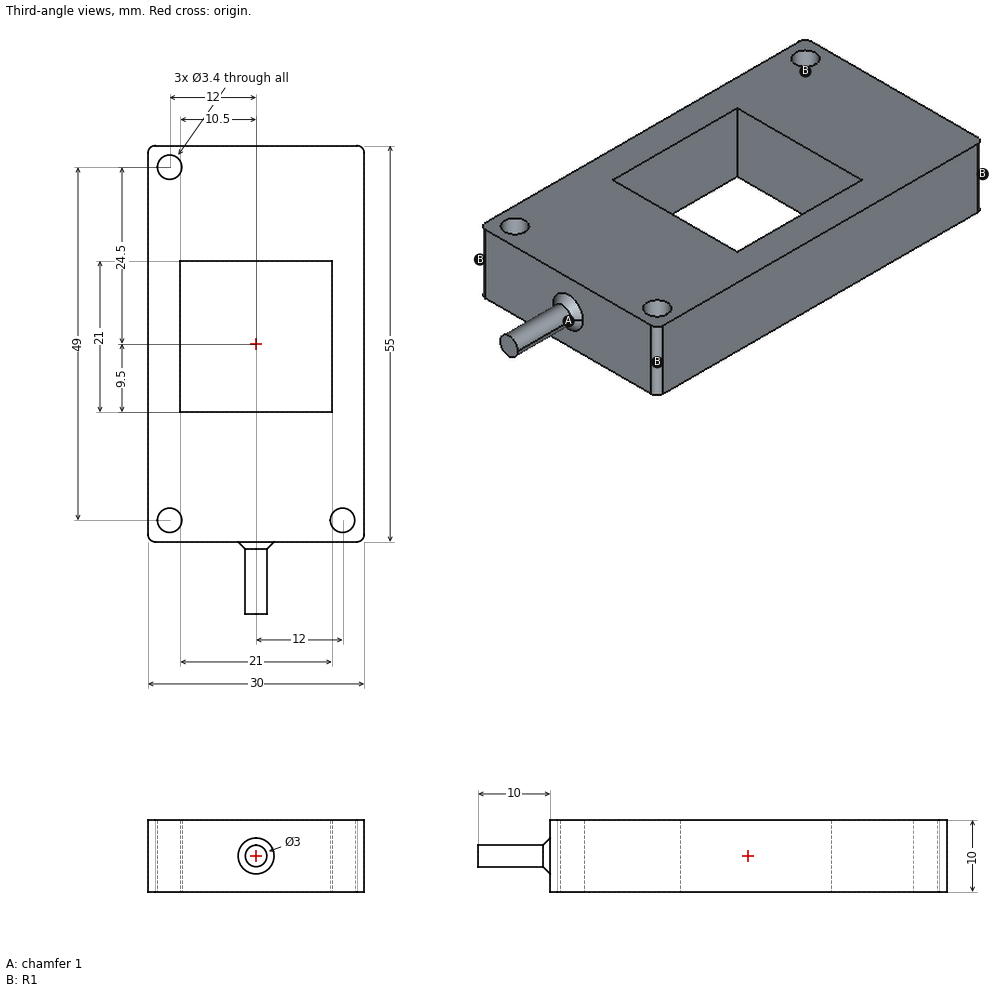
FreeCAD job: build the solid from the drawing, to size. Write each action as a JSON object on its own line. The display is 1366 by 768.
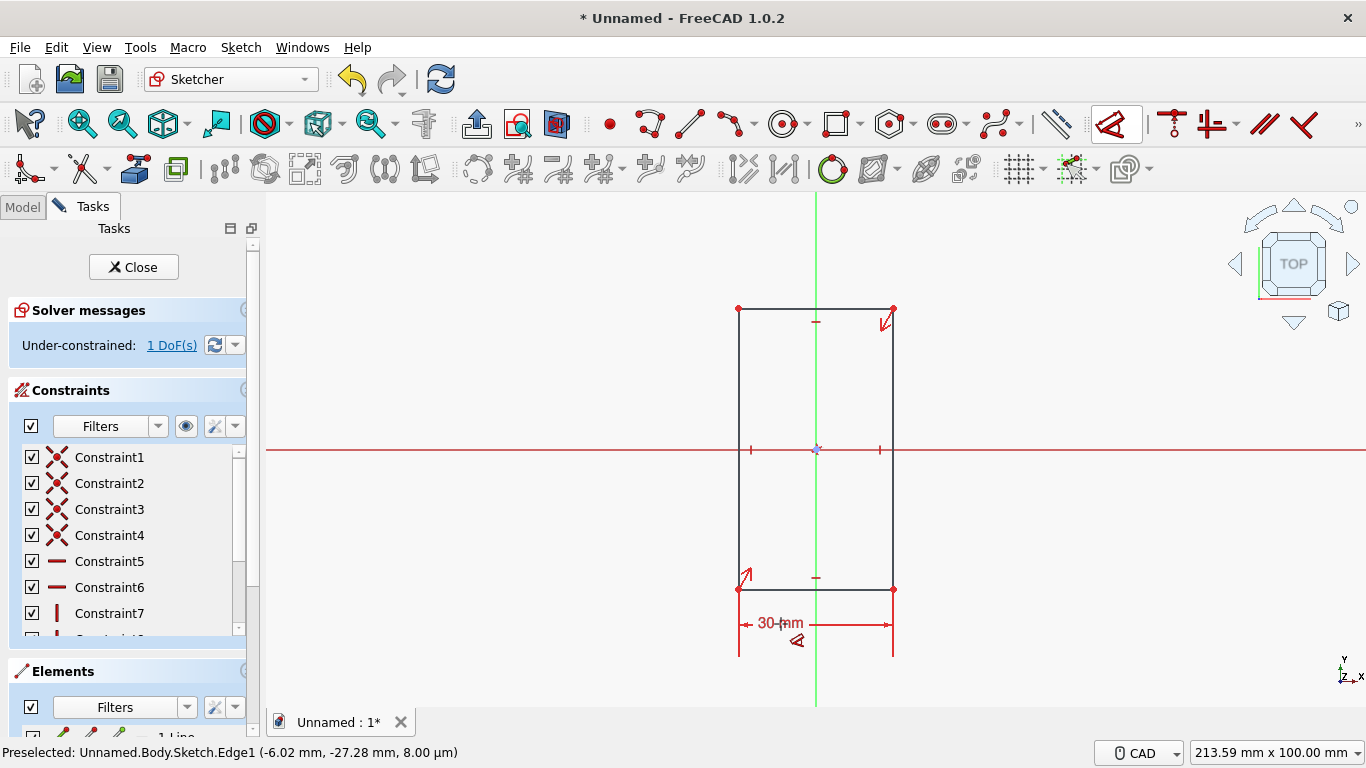
{"action": "left_click", "coordinate": [893, 506]}
{"action": "left_click", "coordinate": [927, 385]}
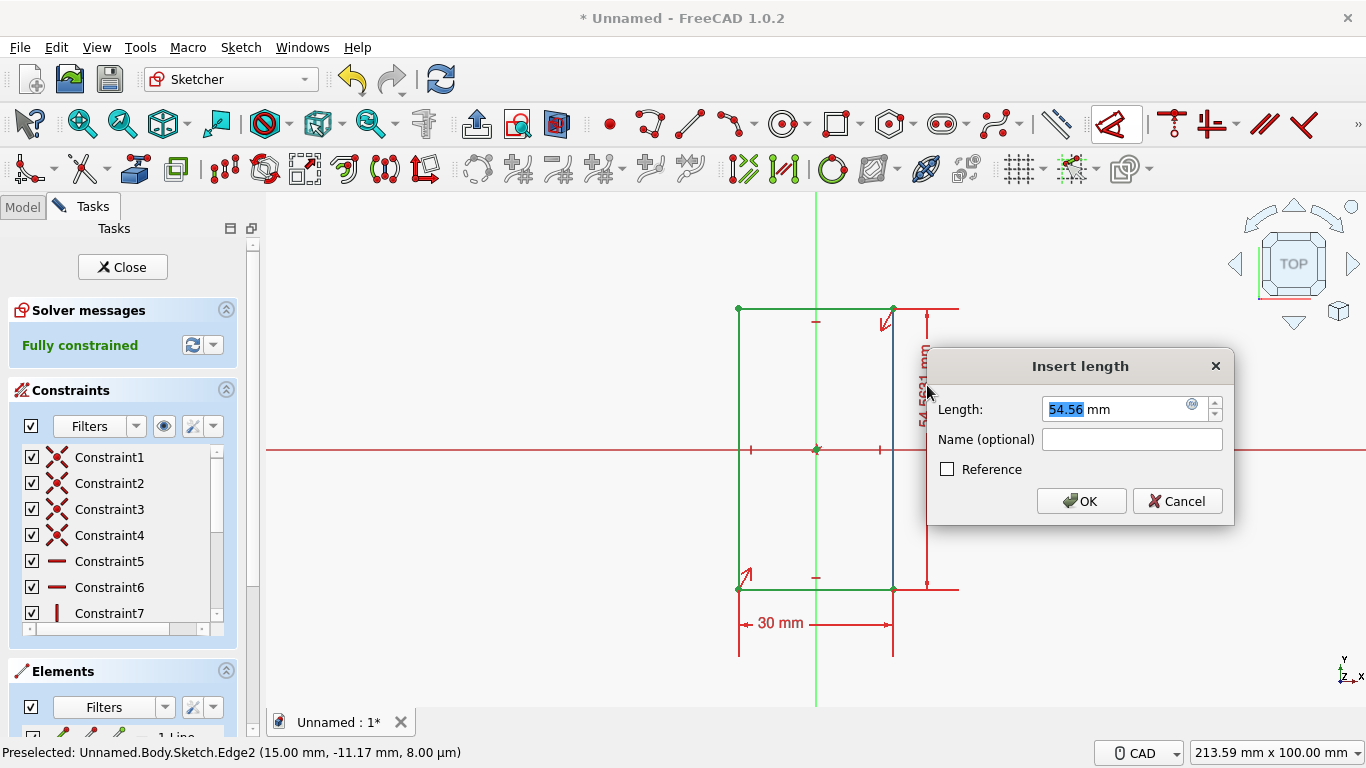
{"action": "type", "text": "55"}
{"action": "key", "text": "Return"}
{"action": "key", "text": "Escape"}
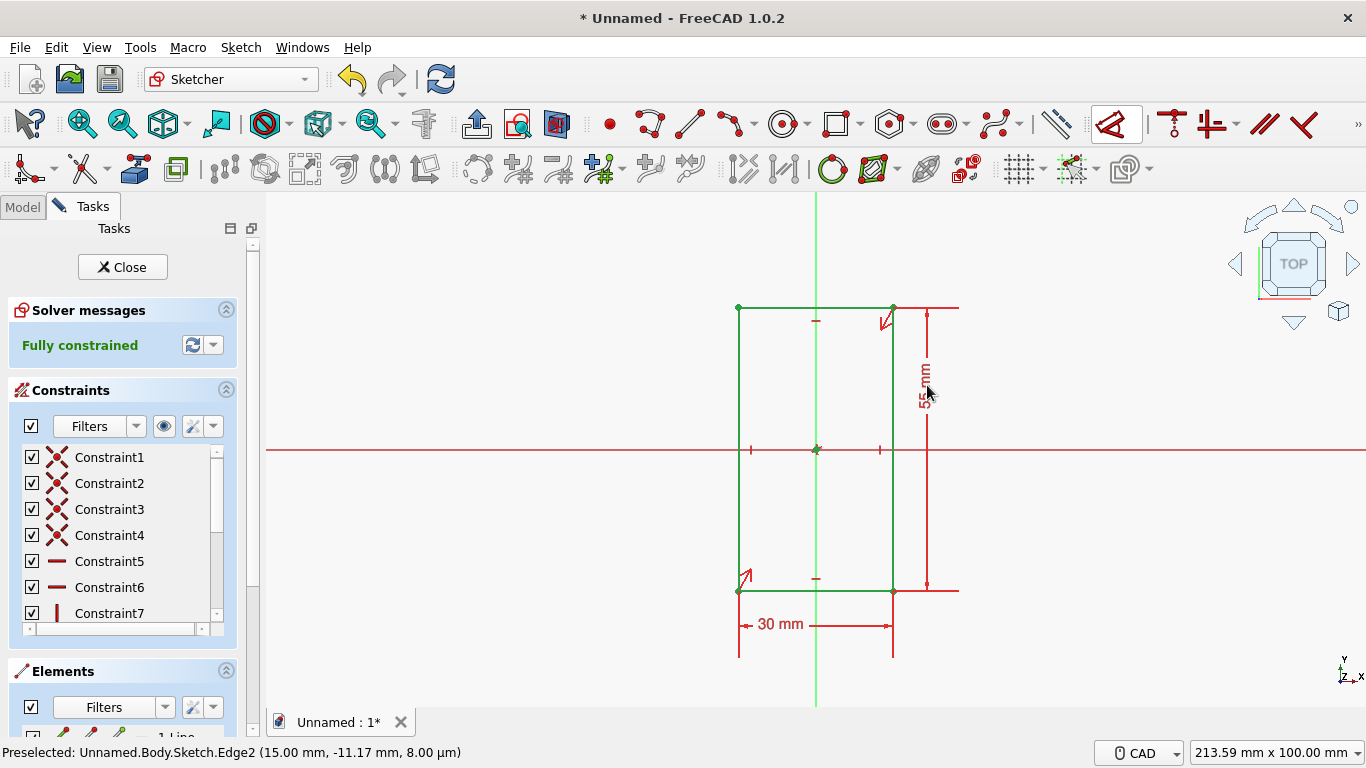
{"action": "left_click", "coordinate": [123, 267]}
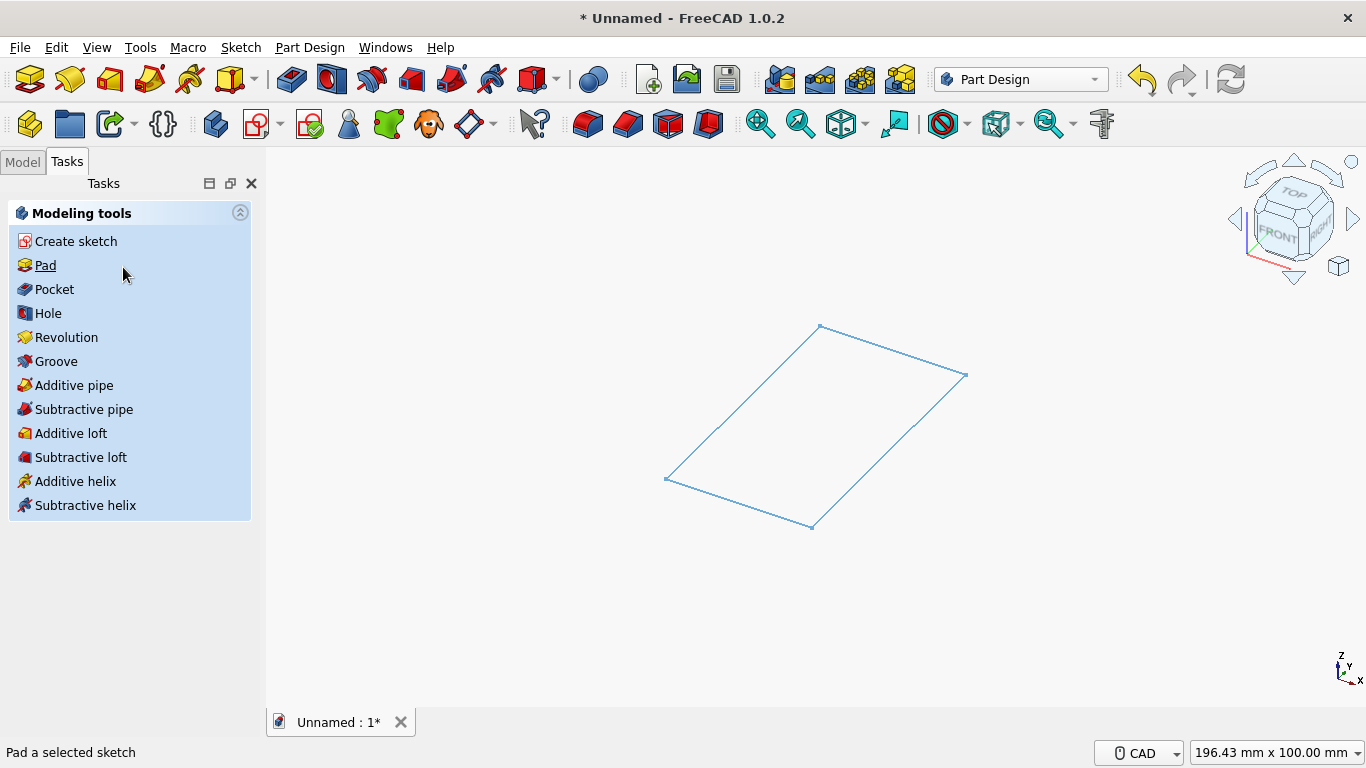
{"action": "left_click", "coordinate": [30, 80]}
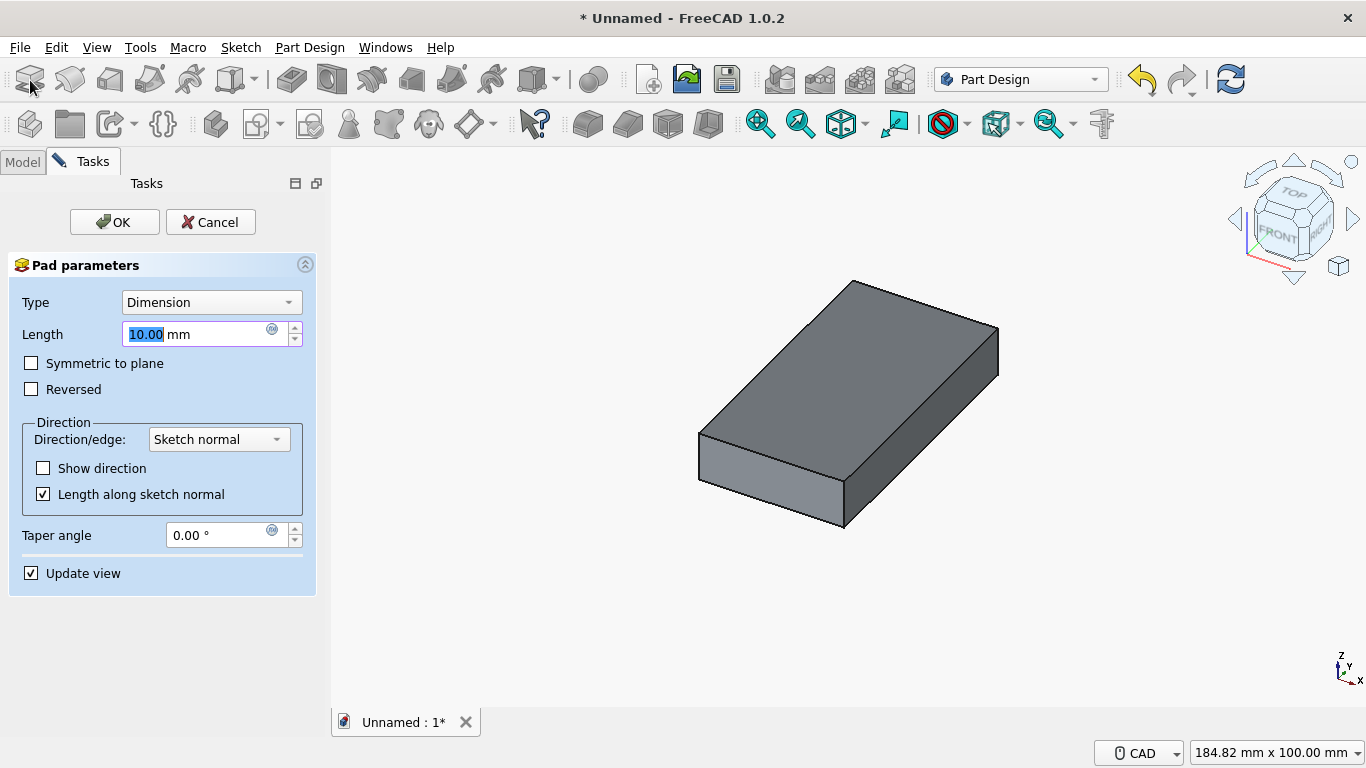
{"action": "type", "text": "10"}
{"action": "key", "text": "Tab"}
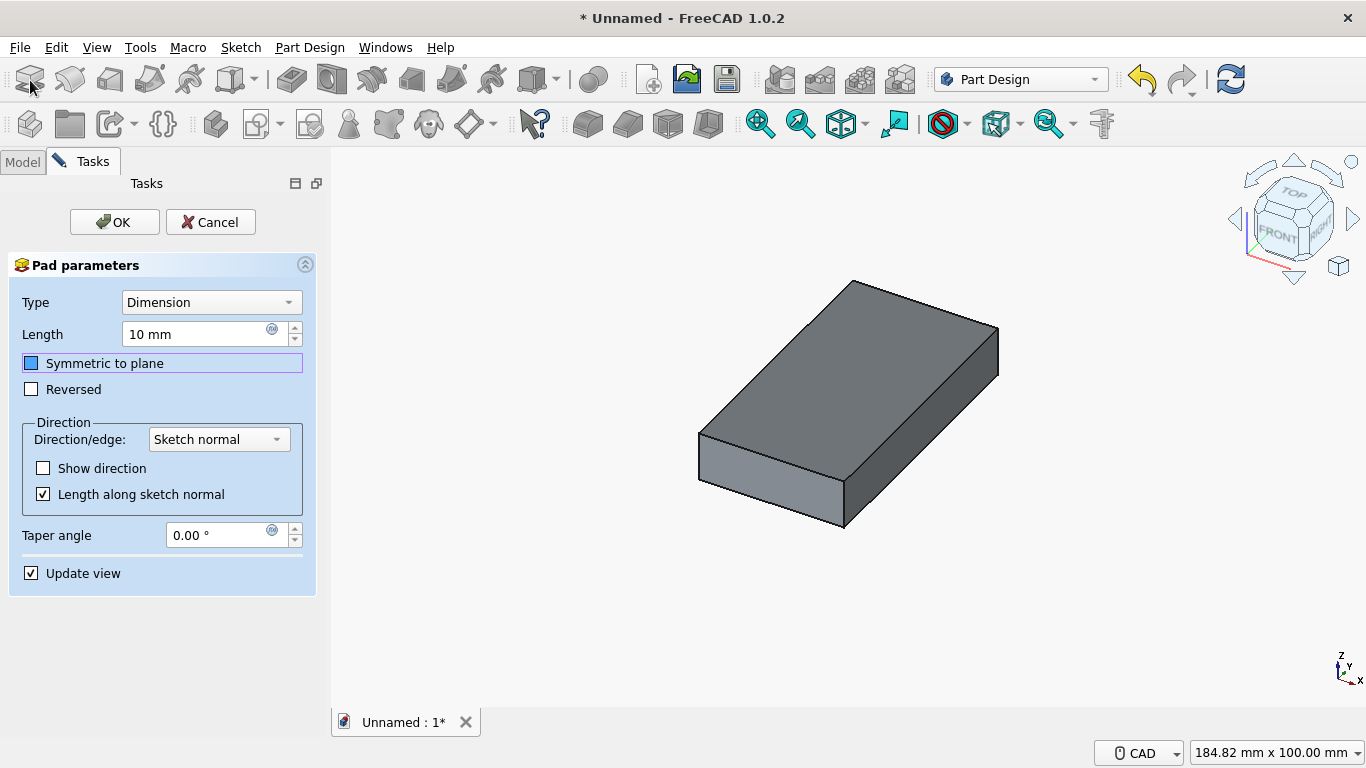
{"action": "left_click", "coordinate": [30, 363]}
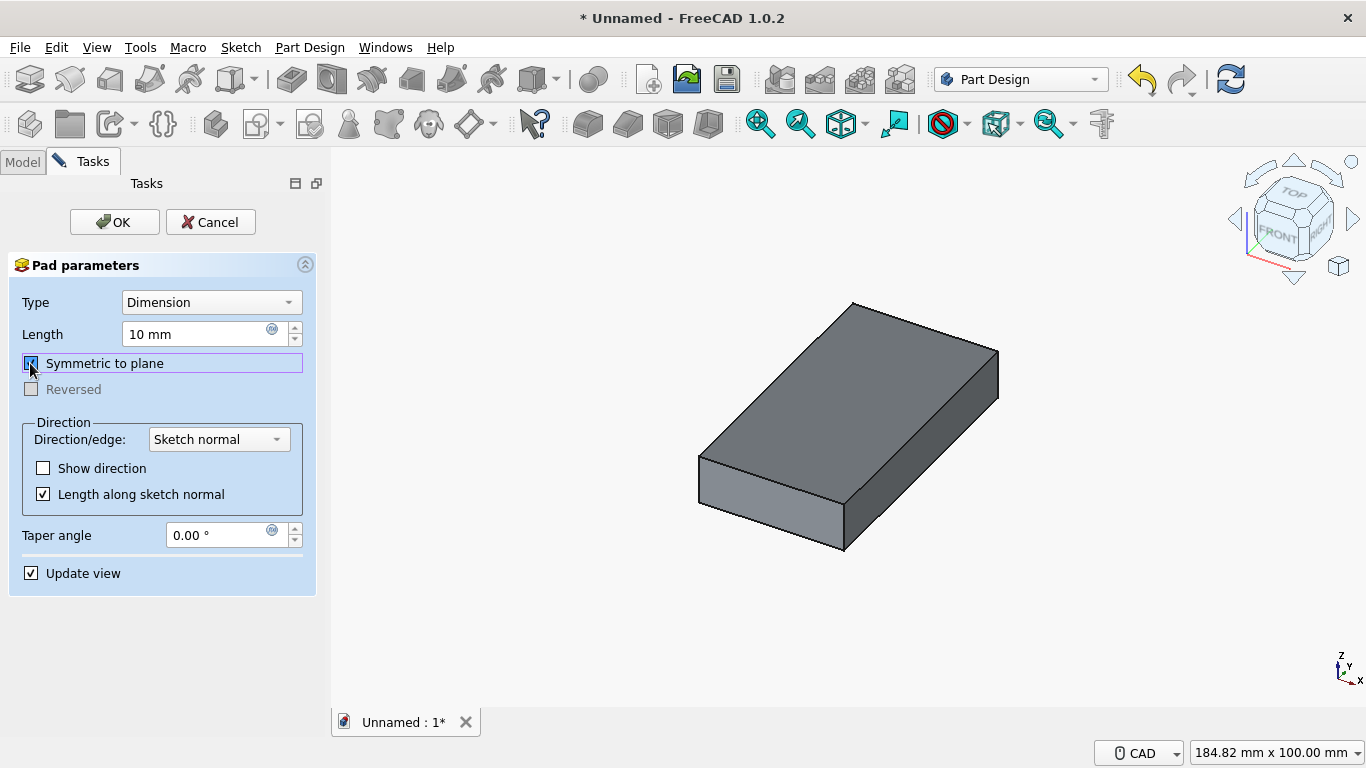
{"action": "left_click", "coordinate": [115, 222]}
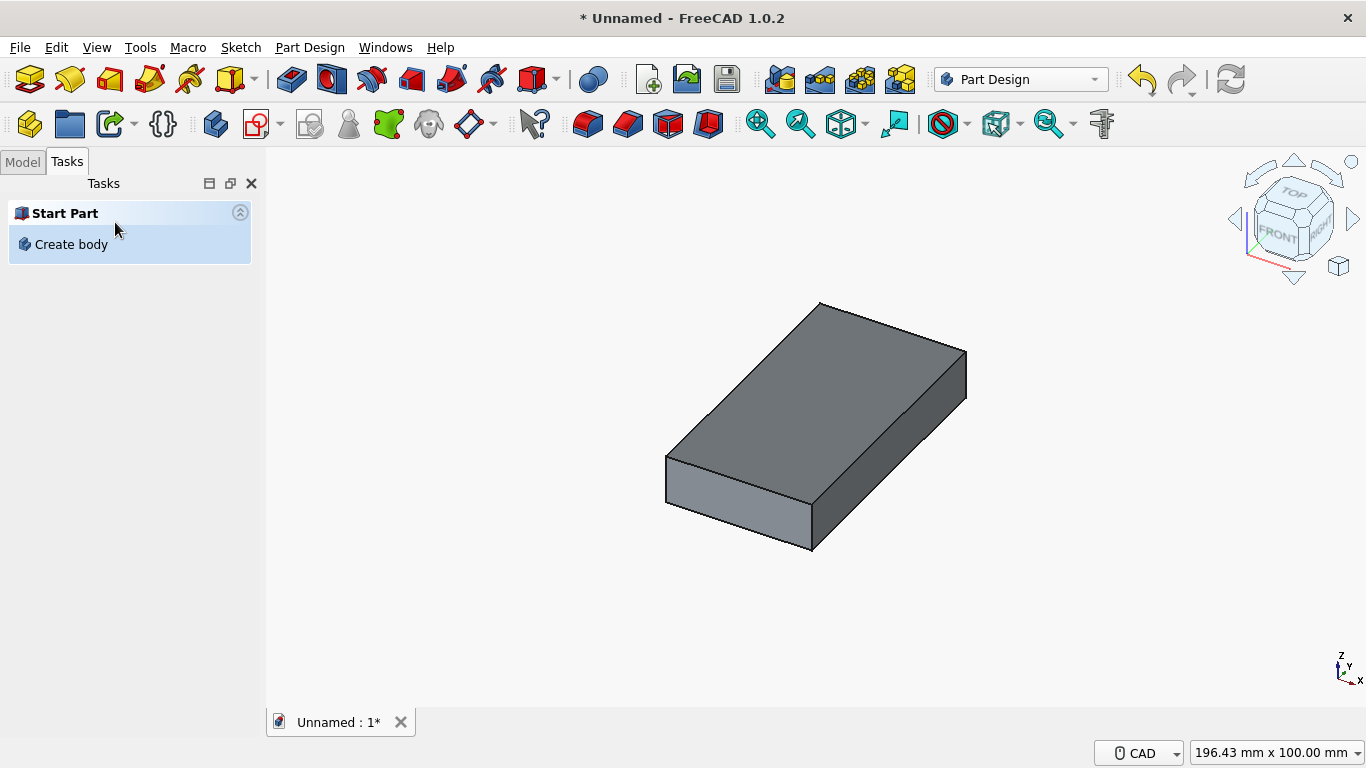
{"action": "key", "text": "v f"}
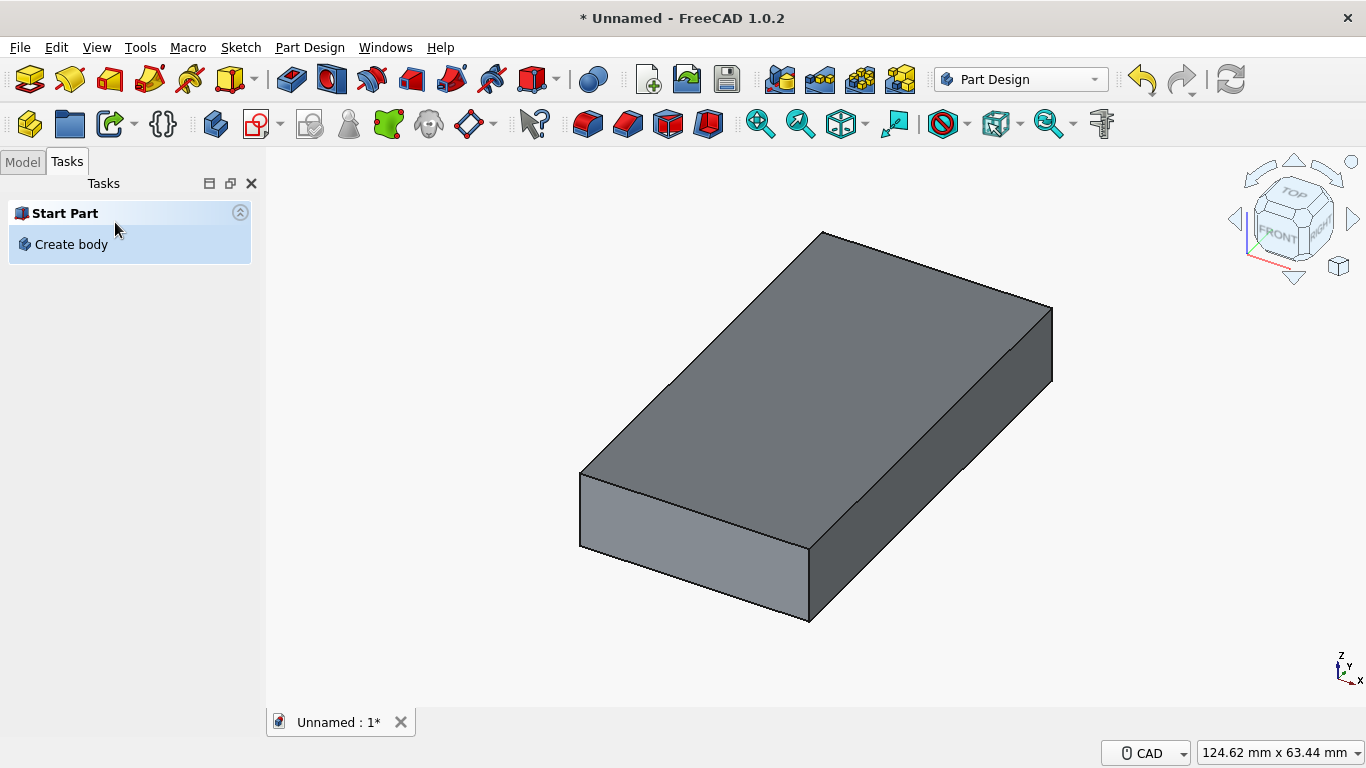
{"action": "left_click", "coordinate": [851, 355]}